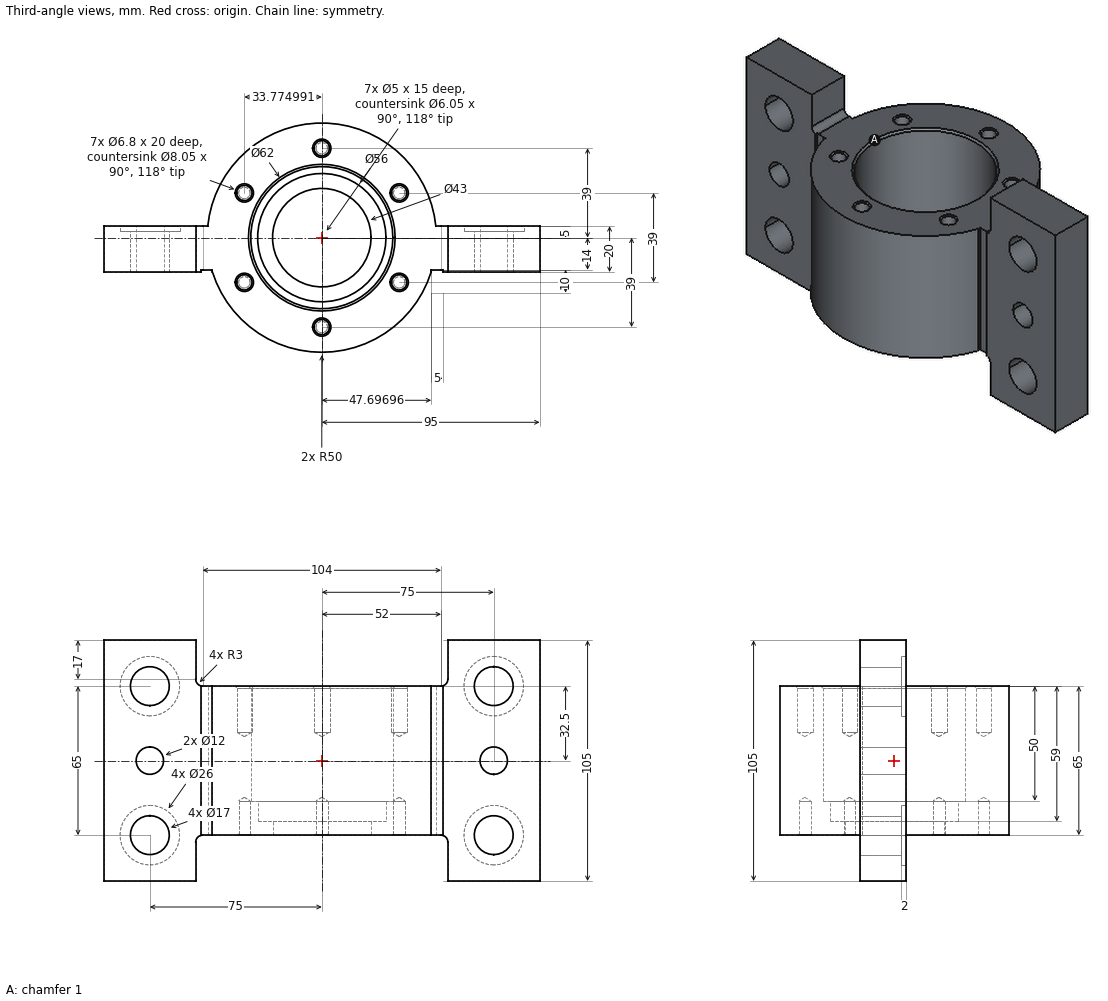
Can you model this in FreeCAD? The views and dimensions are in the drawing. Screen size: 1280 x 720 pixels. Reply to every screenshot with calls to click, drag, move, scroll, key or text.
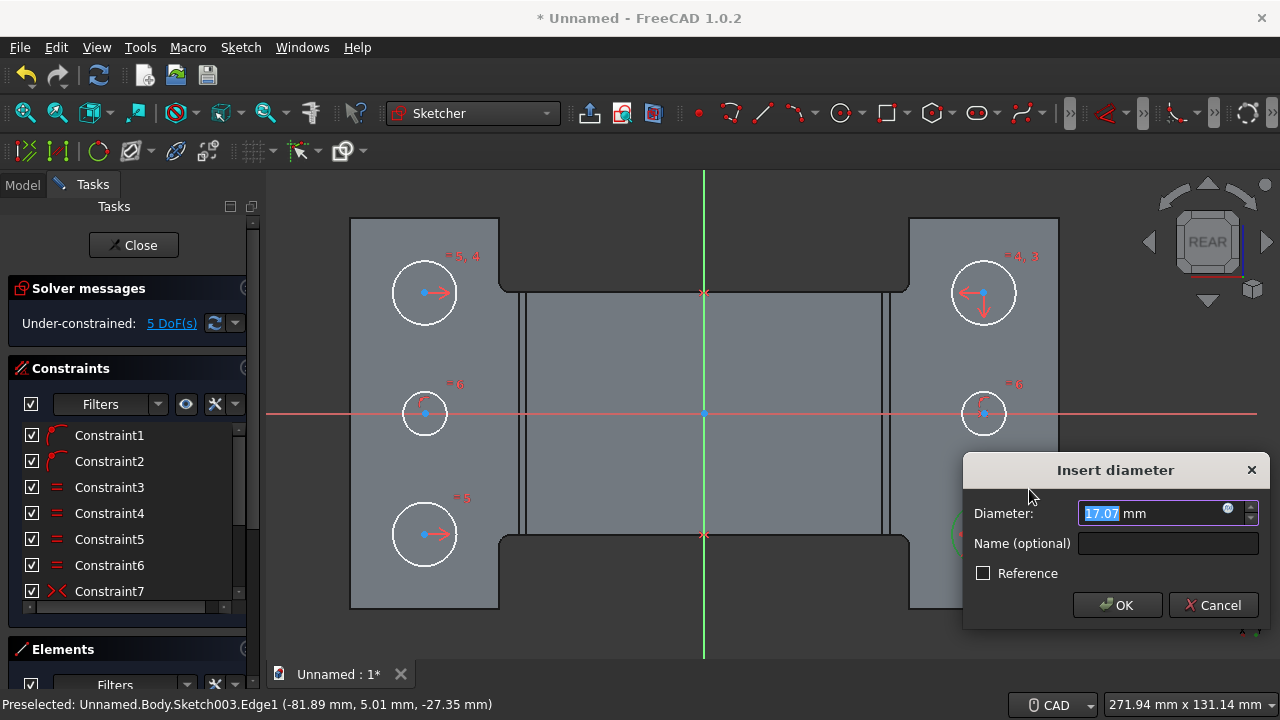
text(17)
key(Return)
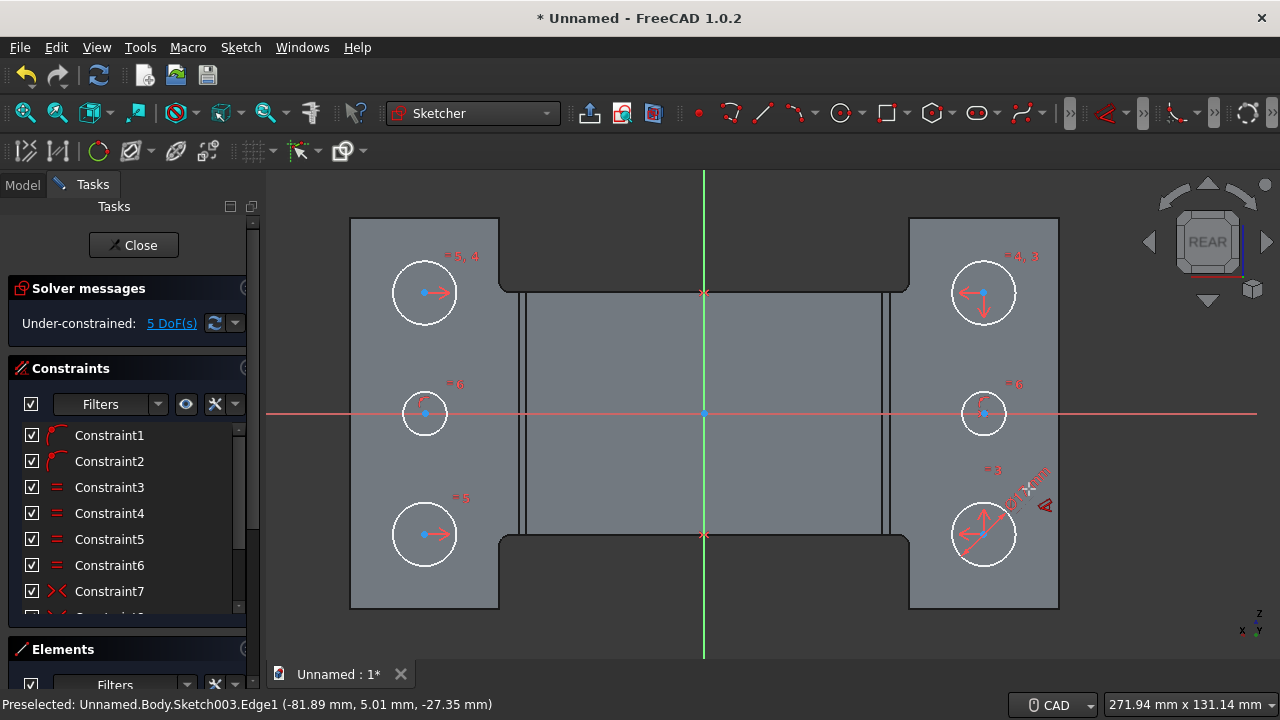
click(999, 398)
click(1021, 375)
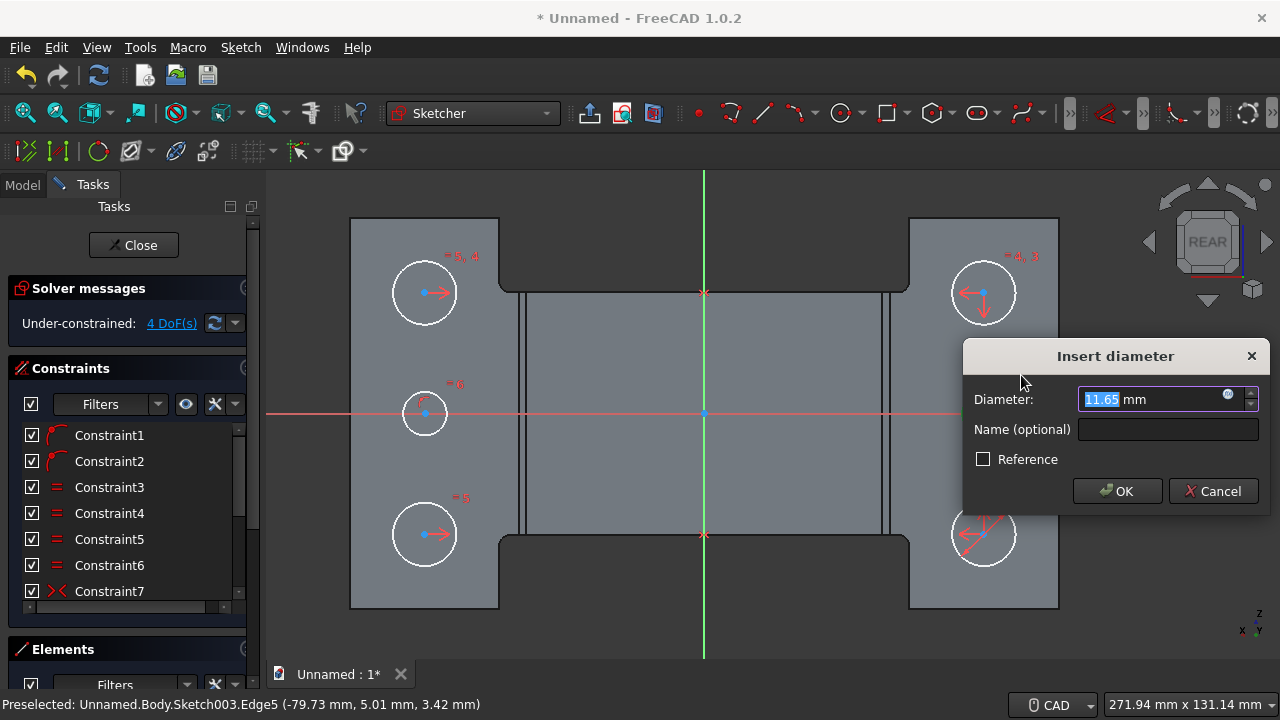
text(12)
key(Return)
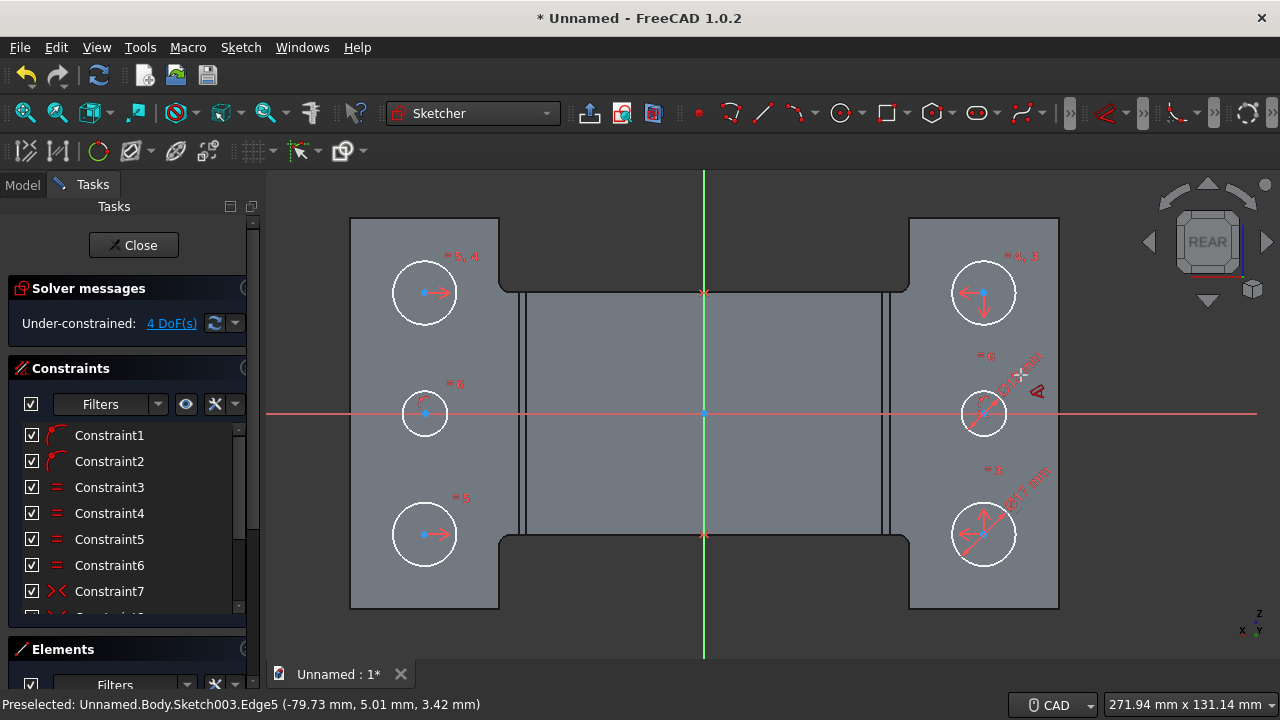
click(984, 534)
click(844, 568)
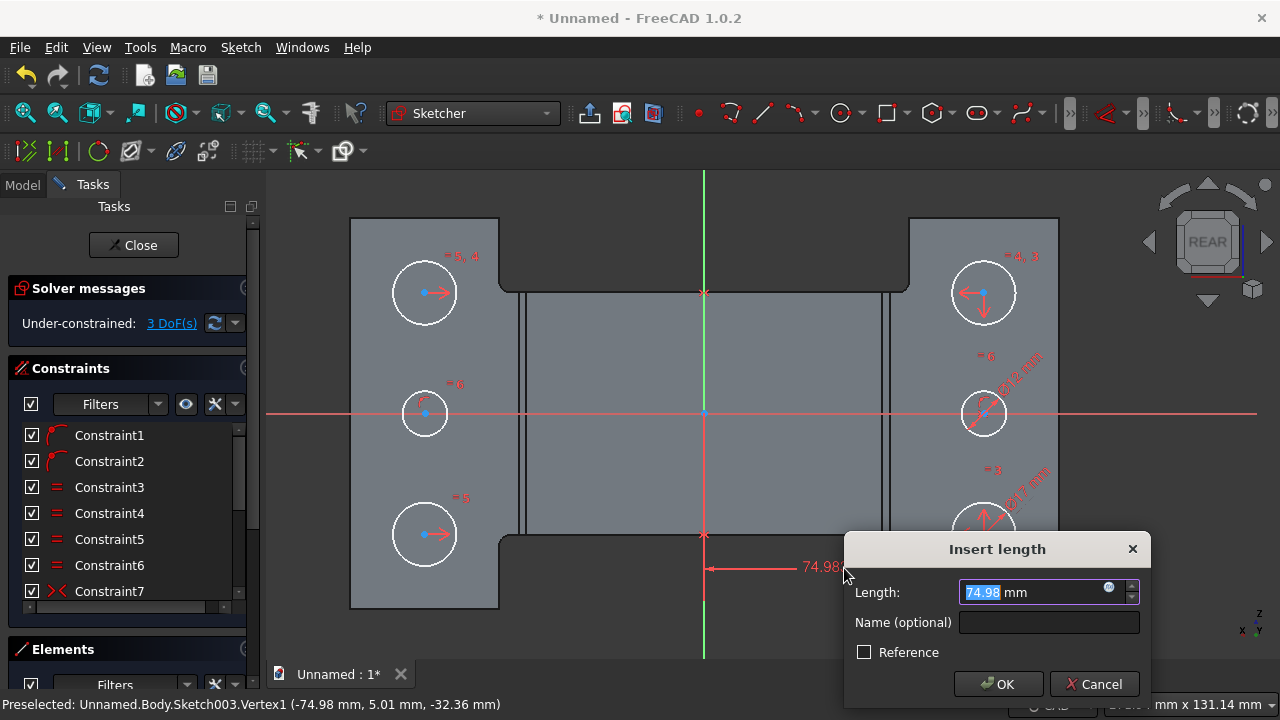
text(75)
key(Return)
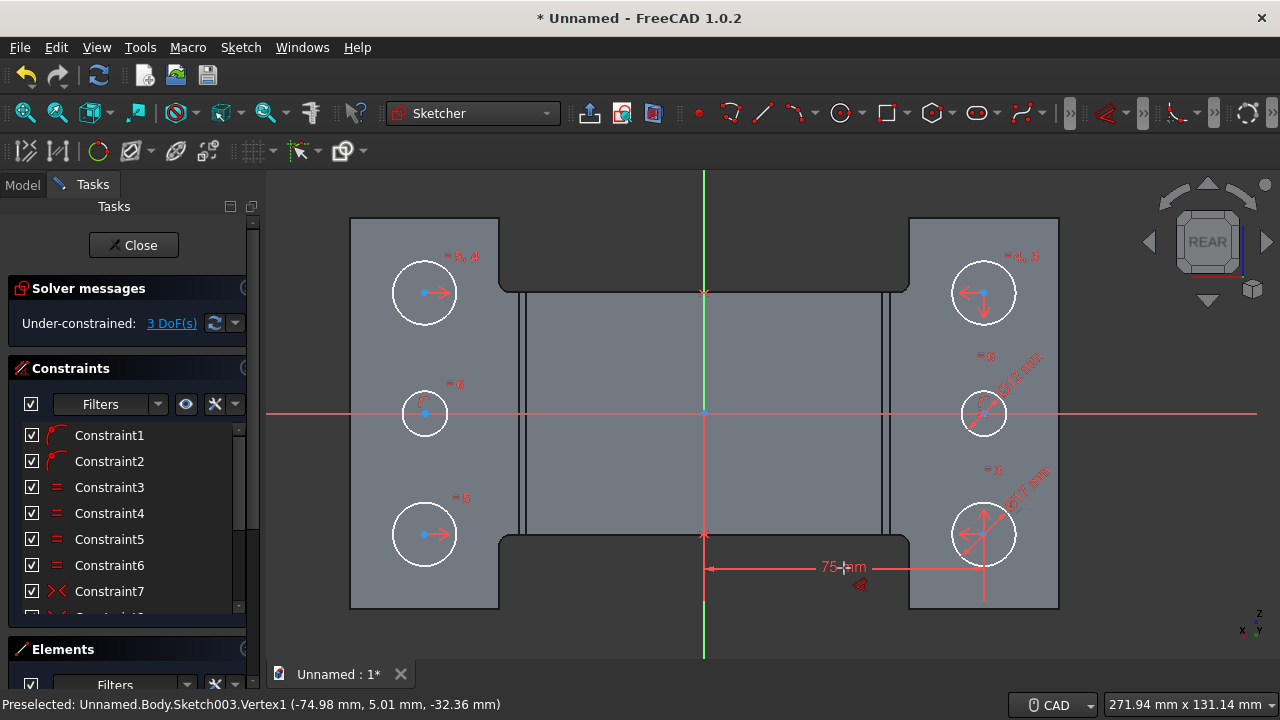
click(984, 414)
click(844, 448)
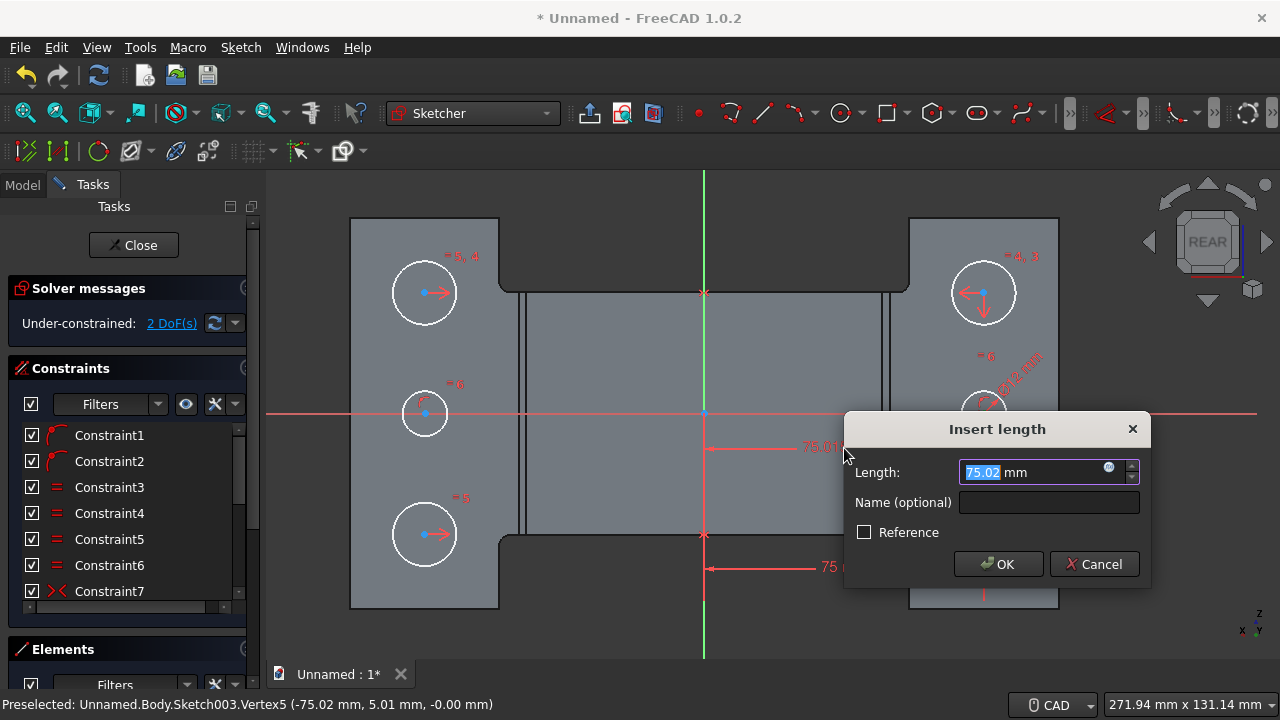
text(75)
key(Return)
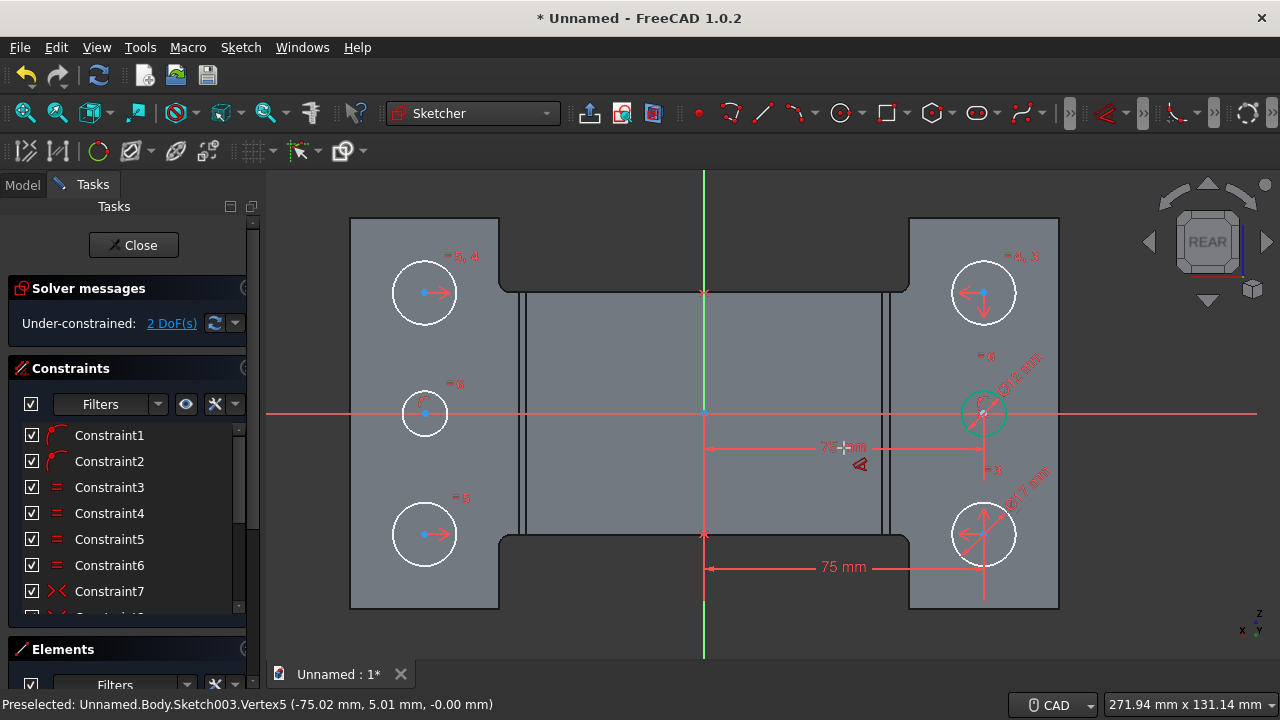
click(425, 414)
click(565, 448)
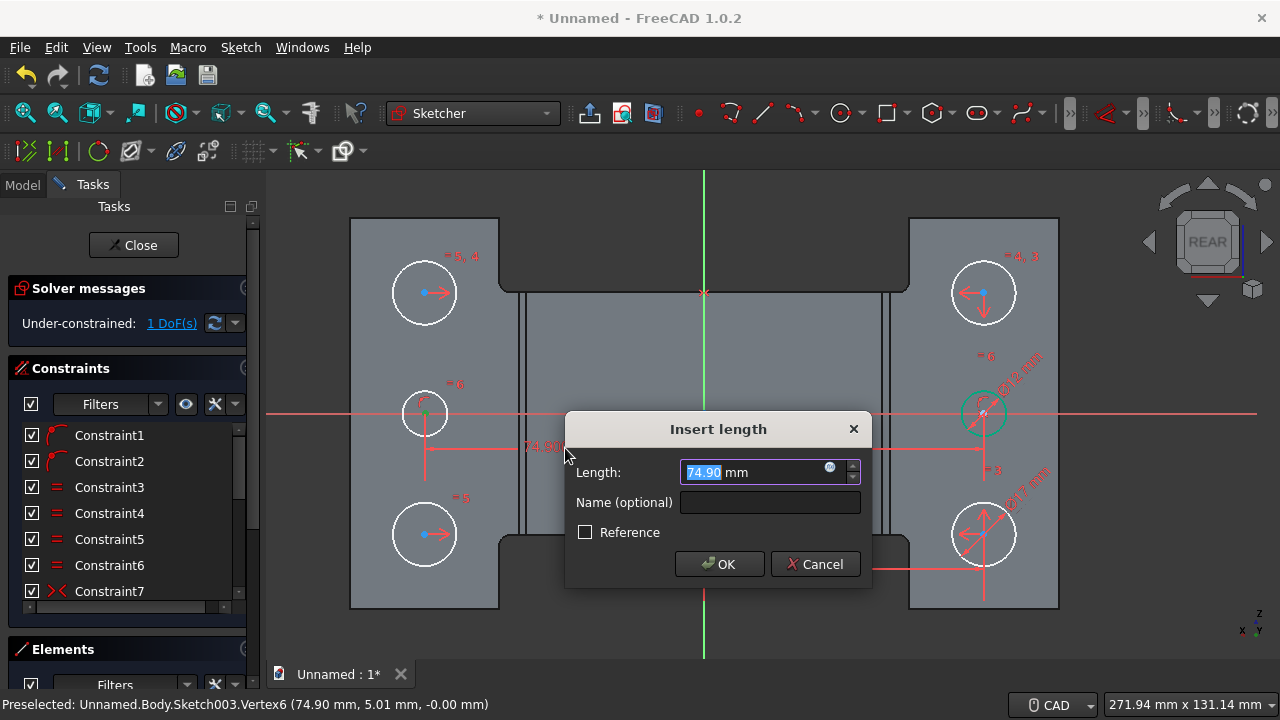
text(75)
key(Return)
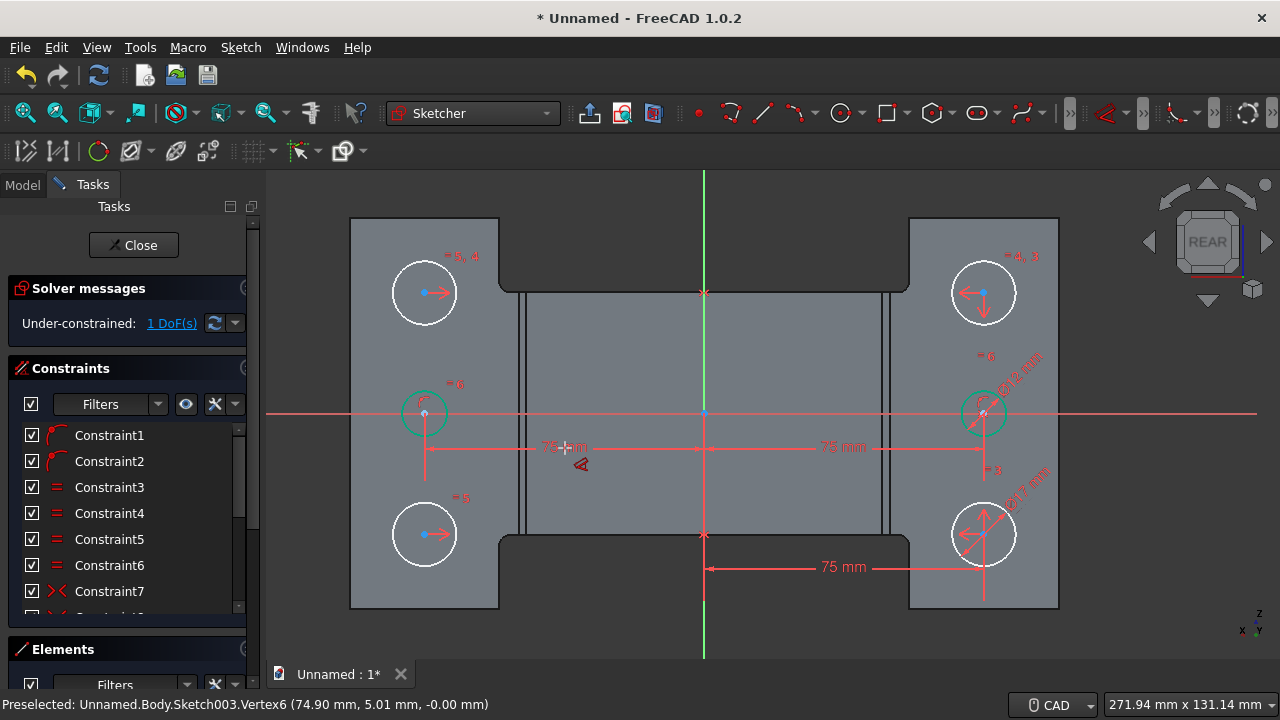
click(984, 534)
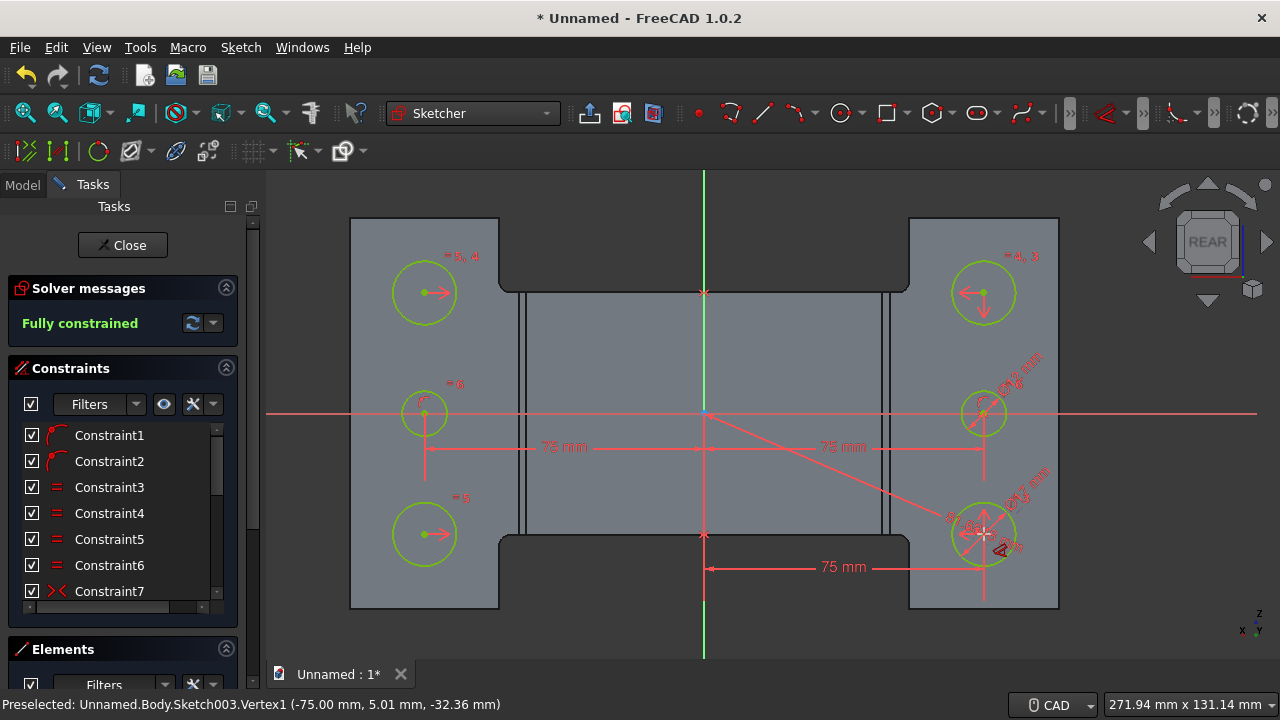
click(984, 293)
click(1018, 469)